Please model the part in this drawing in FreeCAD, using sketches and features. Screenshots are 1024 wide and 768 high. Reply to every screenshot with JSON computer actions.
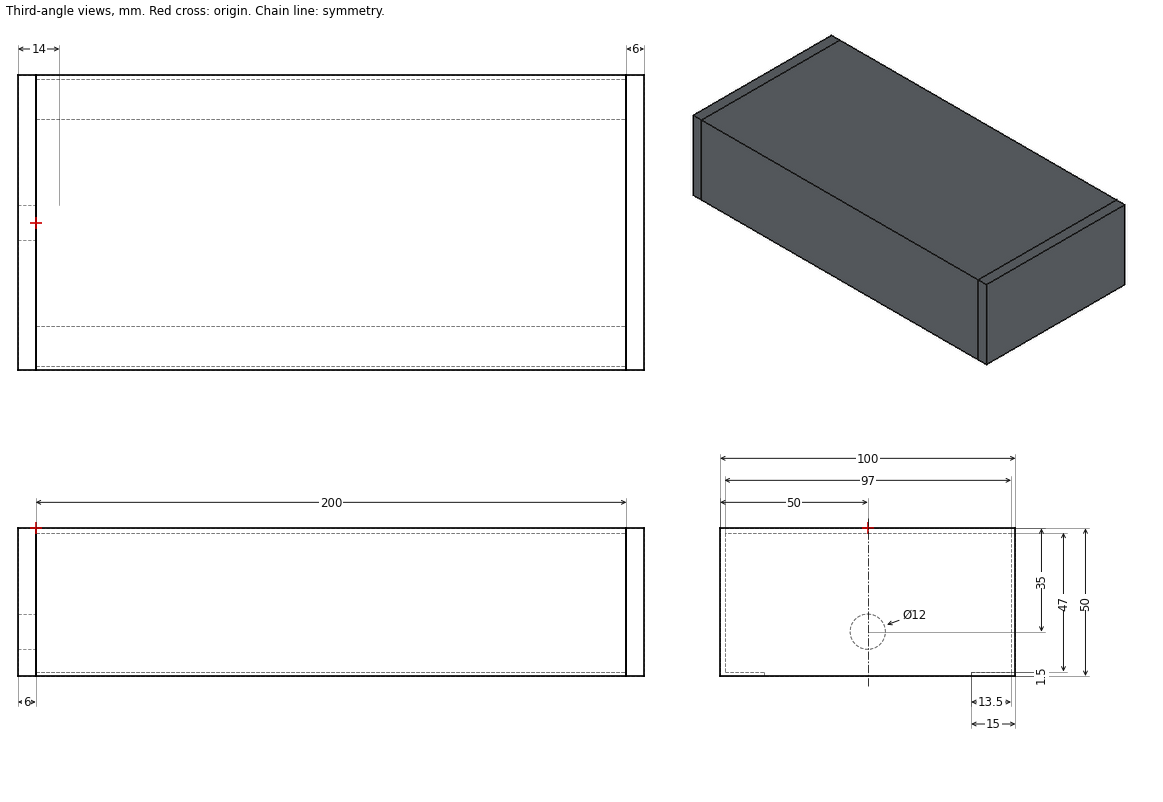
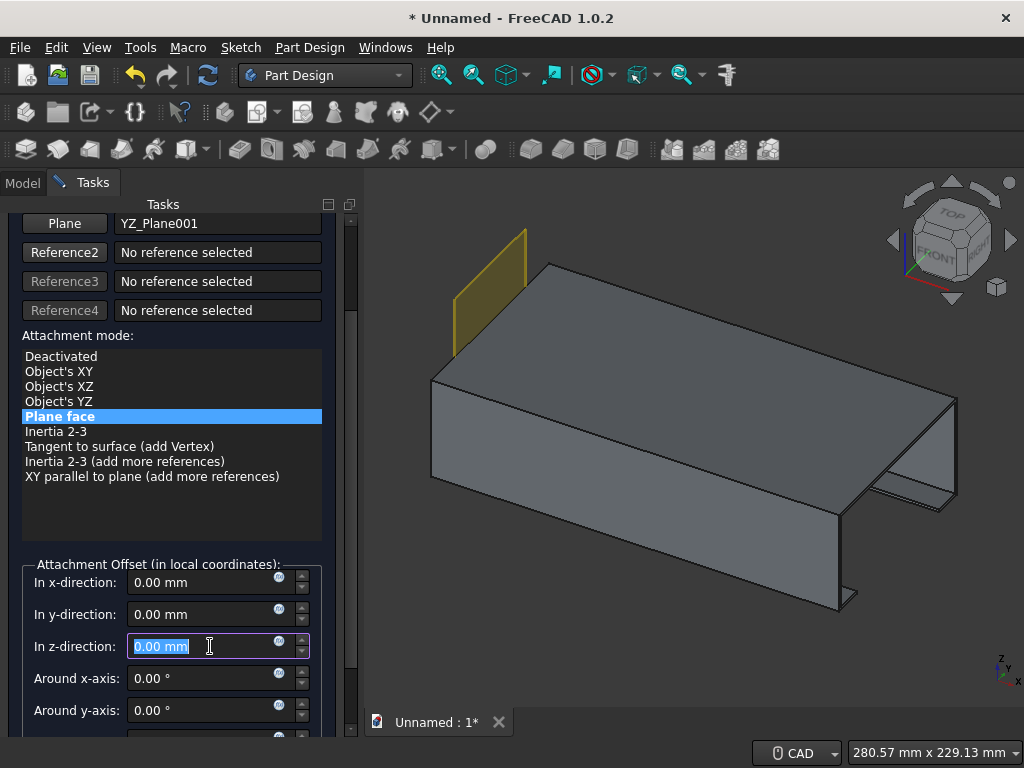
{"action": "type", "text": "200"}
{"action": "key", "text": "Tab"}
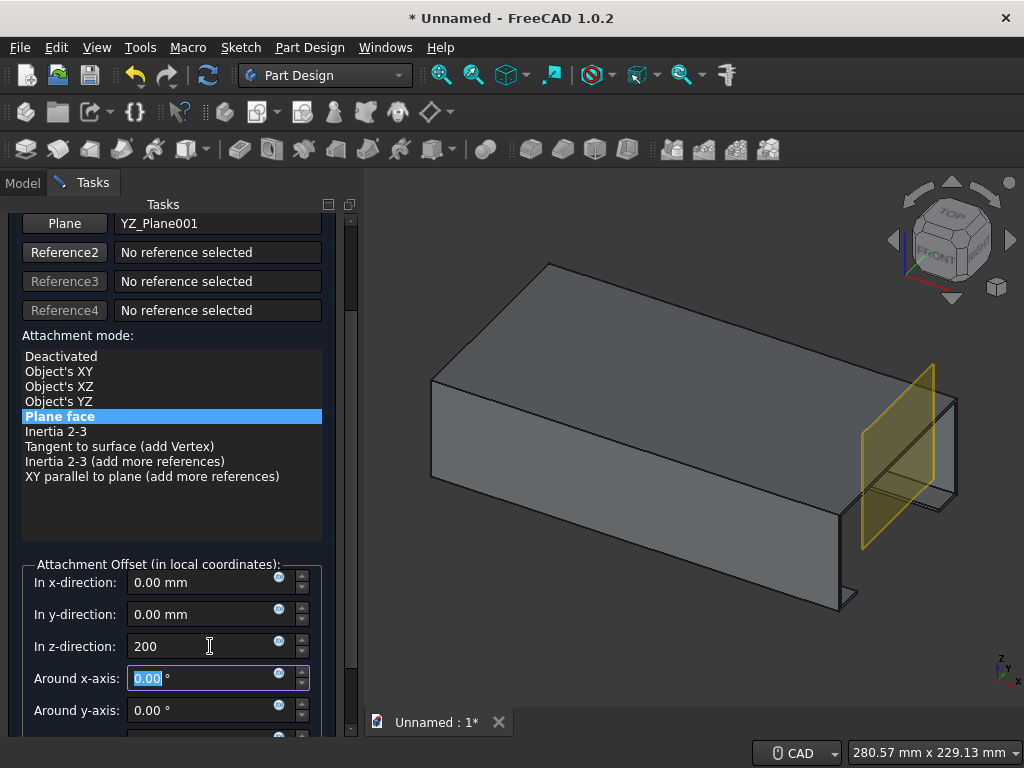
{"action": "scroll", "coordinate": [351, 475], "scroll_direction": "up", "scroll_amount": 3}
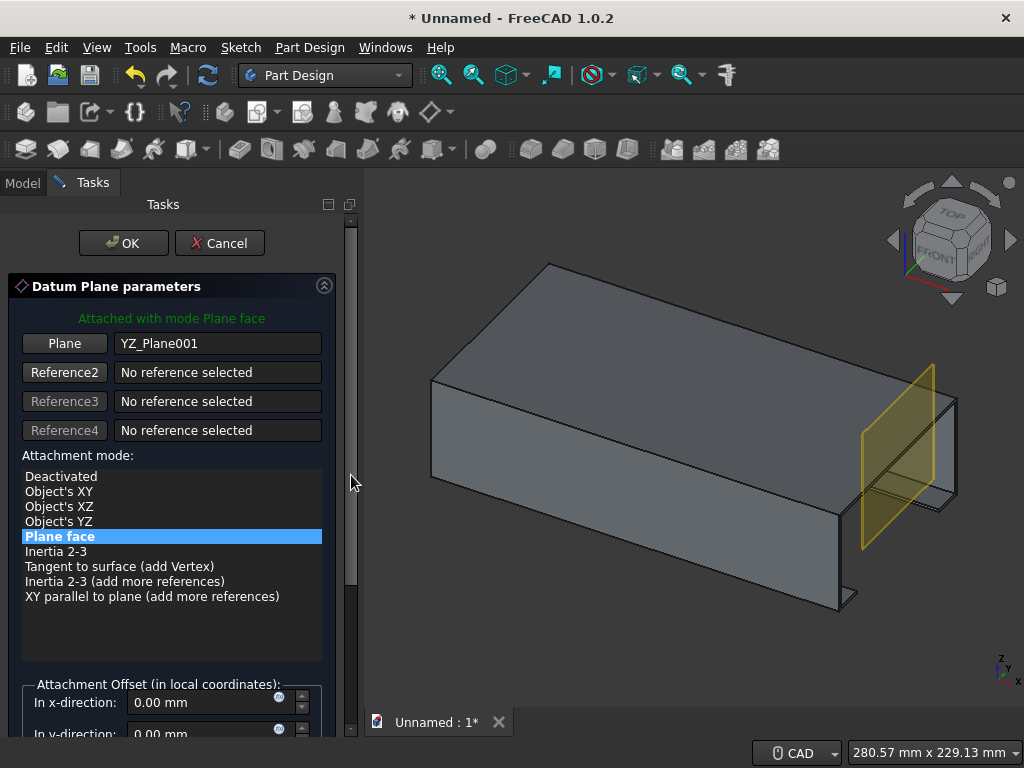
{"action": "left_click", "coordinate": [124, 243]}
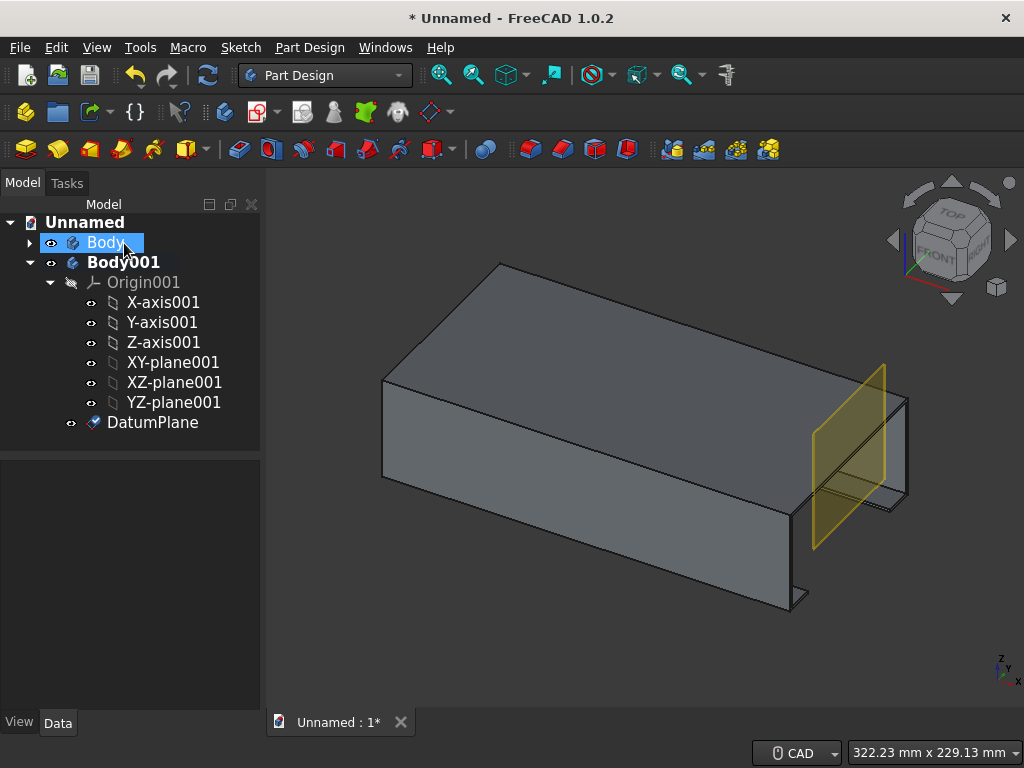
{"action": "left_click", "coordinate": [116, 423]}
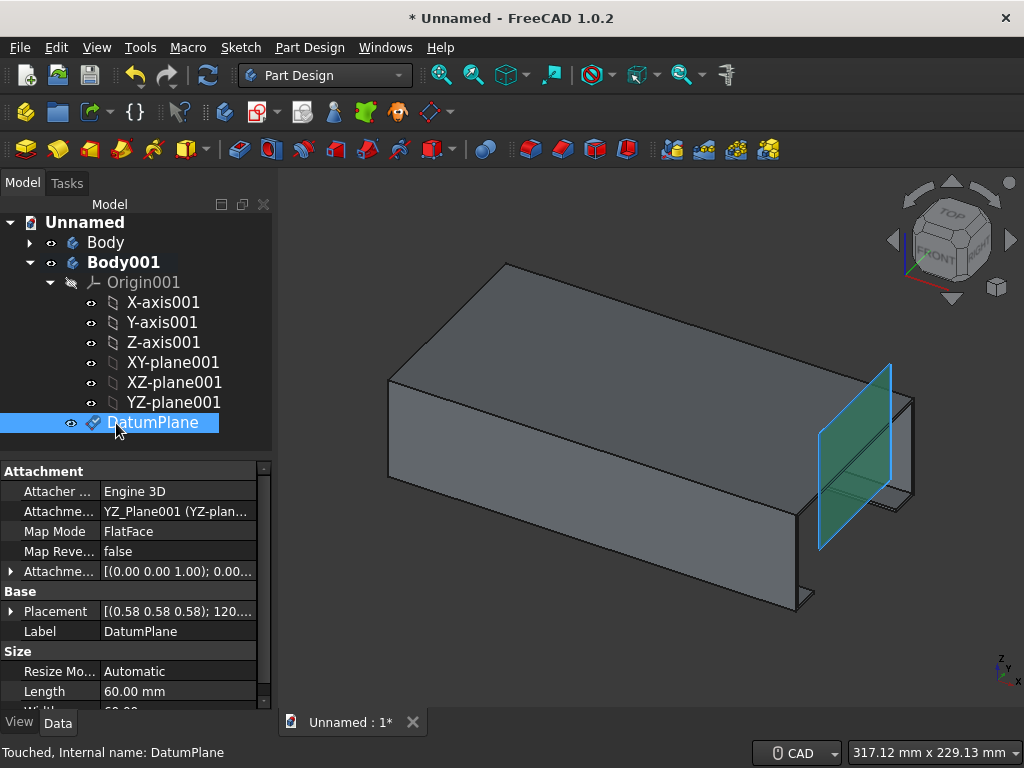
{"action": "left_click", "coordinate": [258, 112]}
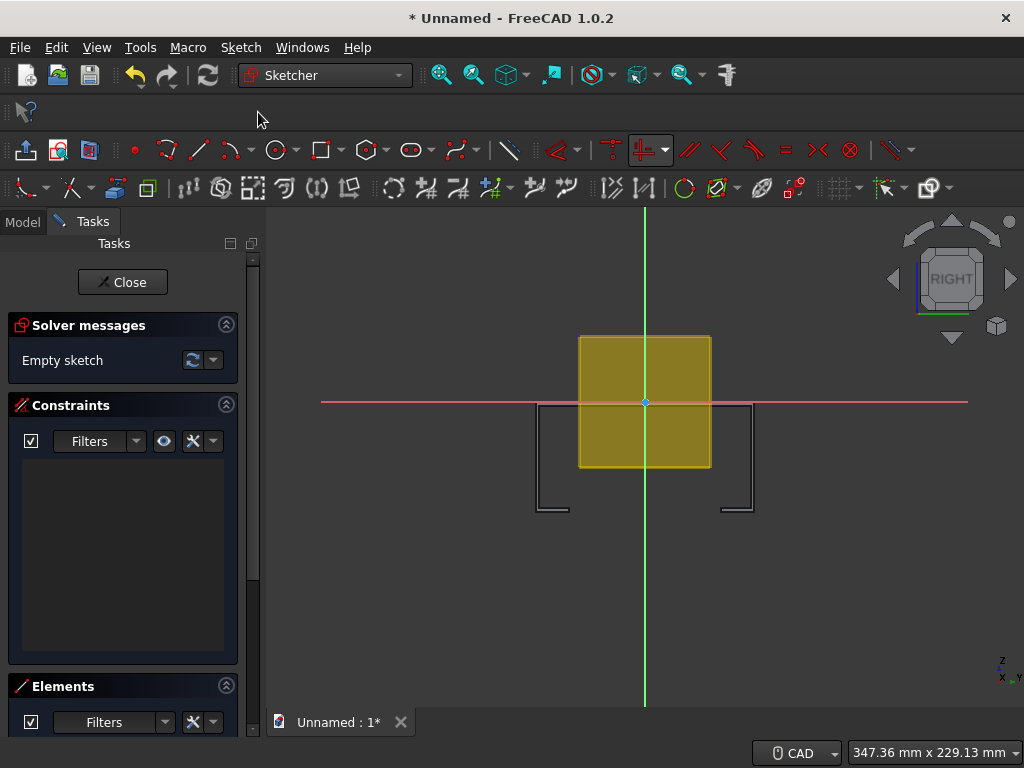
{"action": "scroll", "coordinate": [728, 457], "scroll_direction": "up", "scroll_amount": 3}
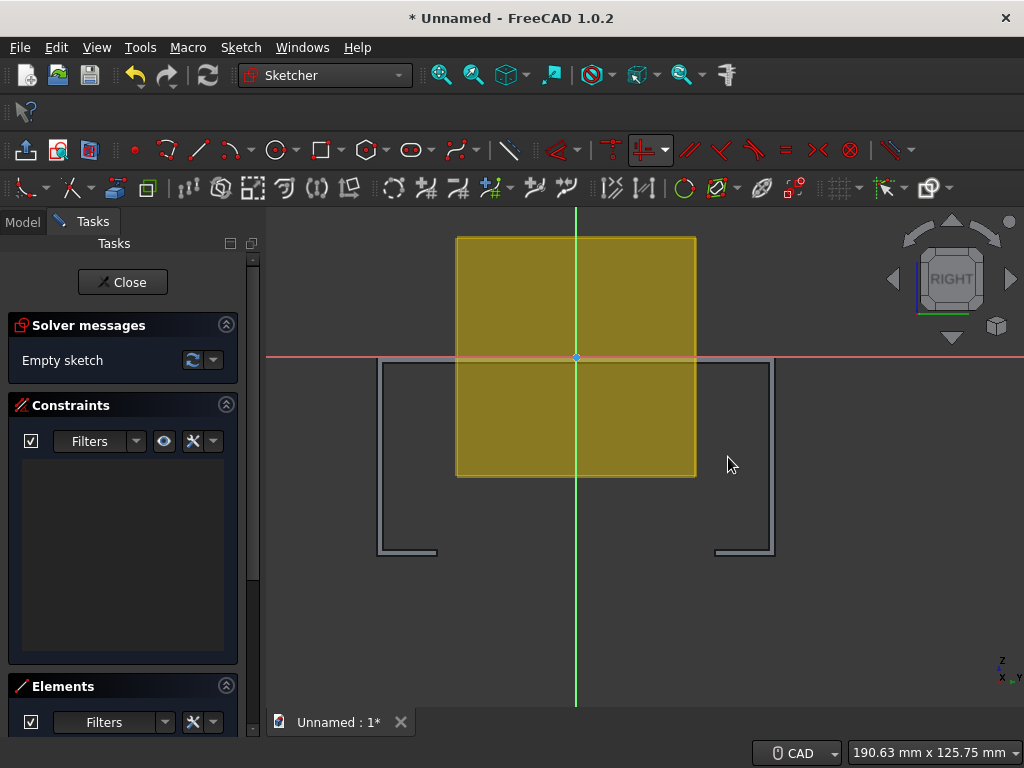
{"action": "left_click", "coordinate": [322, 150]}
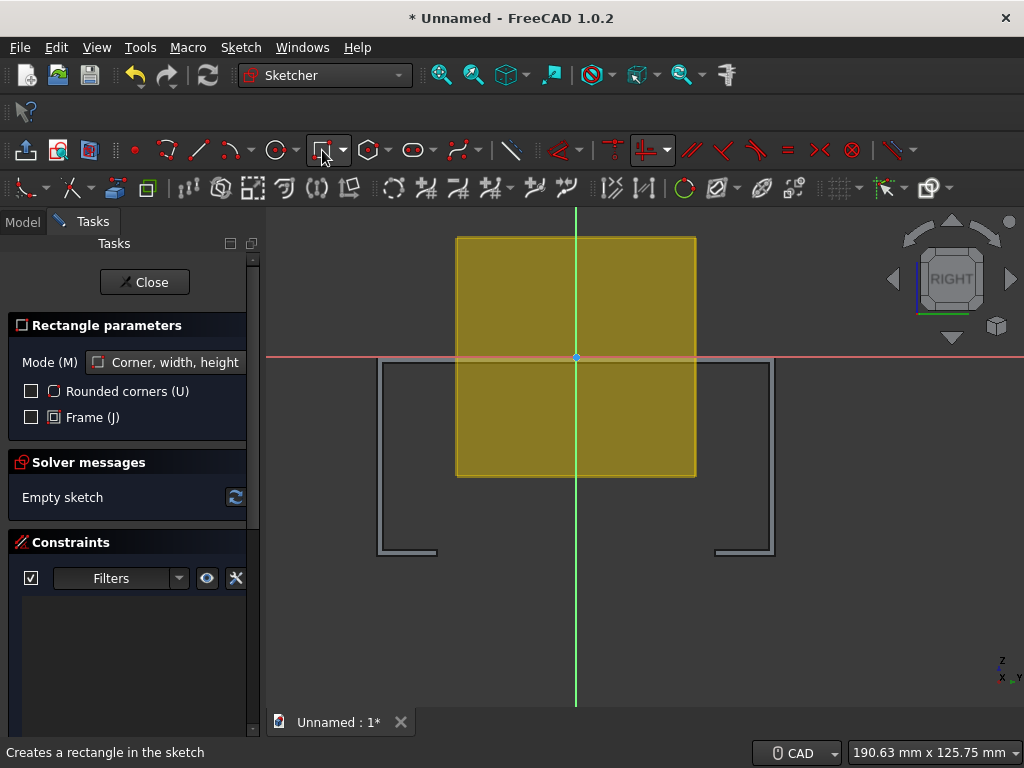
{"action": "left_click", "coordinate": [377, 357]}
{"action": "mouse_move", "coordinate": [775, 556]}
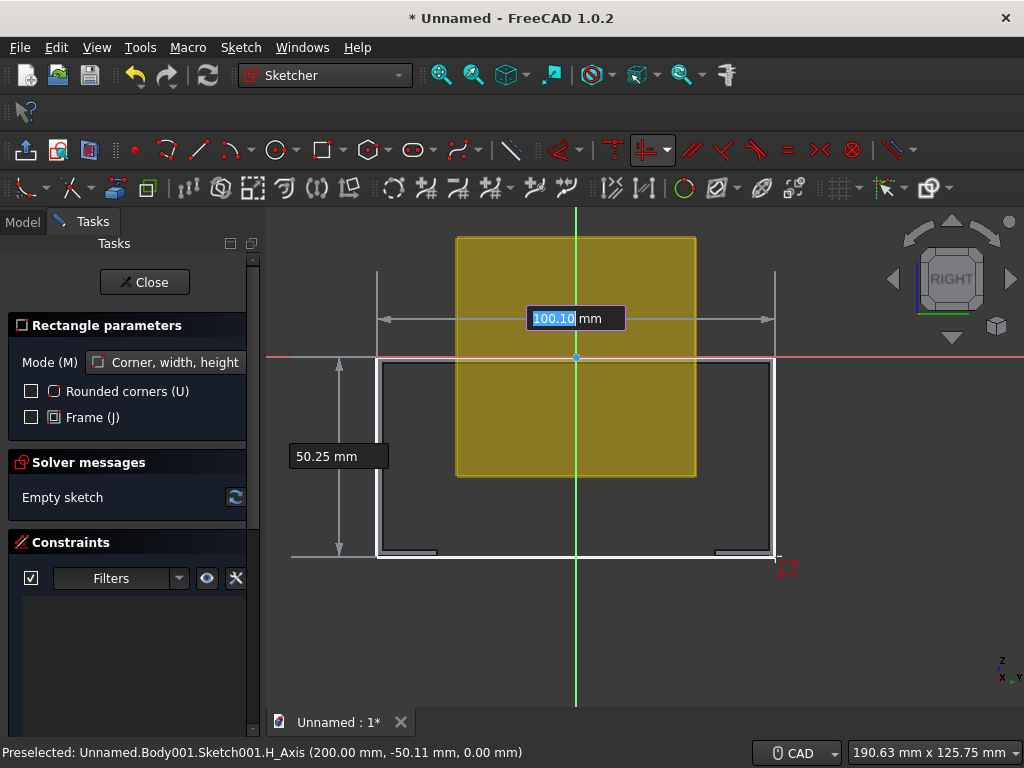
{"action": "type", "text": "100"}
{"action": "key", "text": "Tab"}
{"action": "type", "text": "50"}
{"action": "key", "text": "Return"}
{"action": "key", "text": "Escape"}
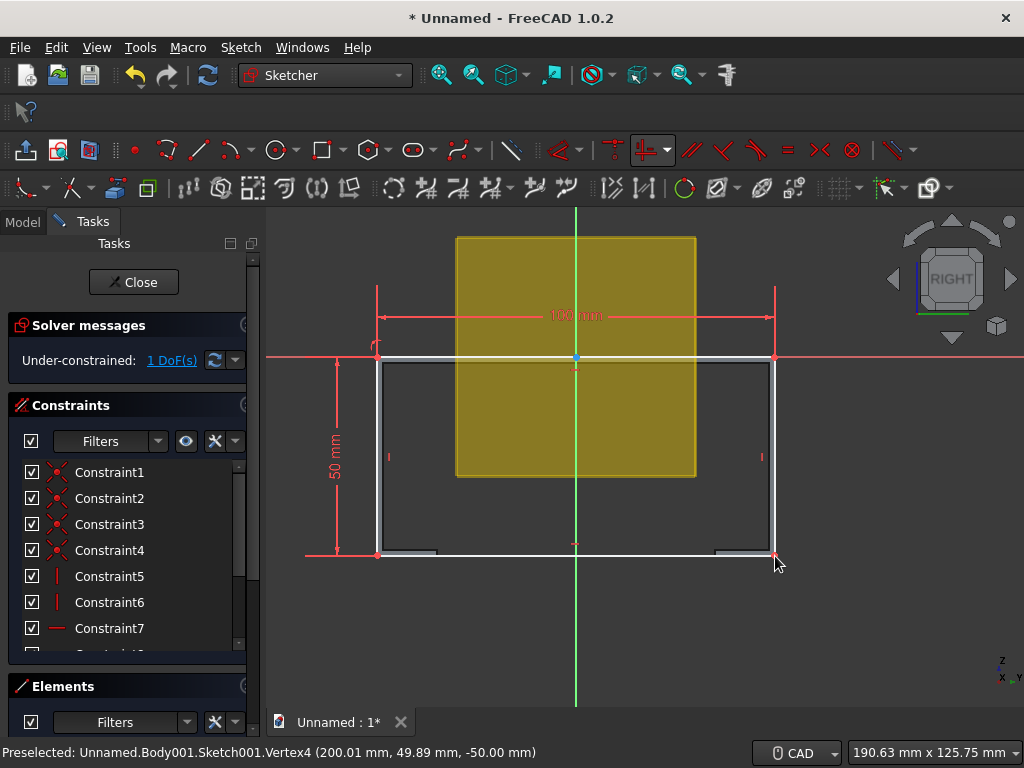
{"action": "left_click", "coordinate": [558, 150]}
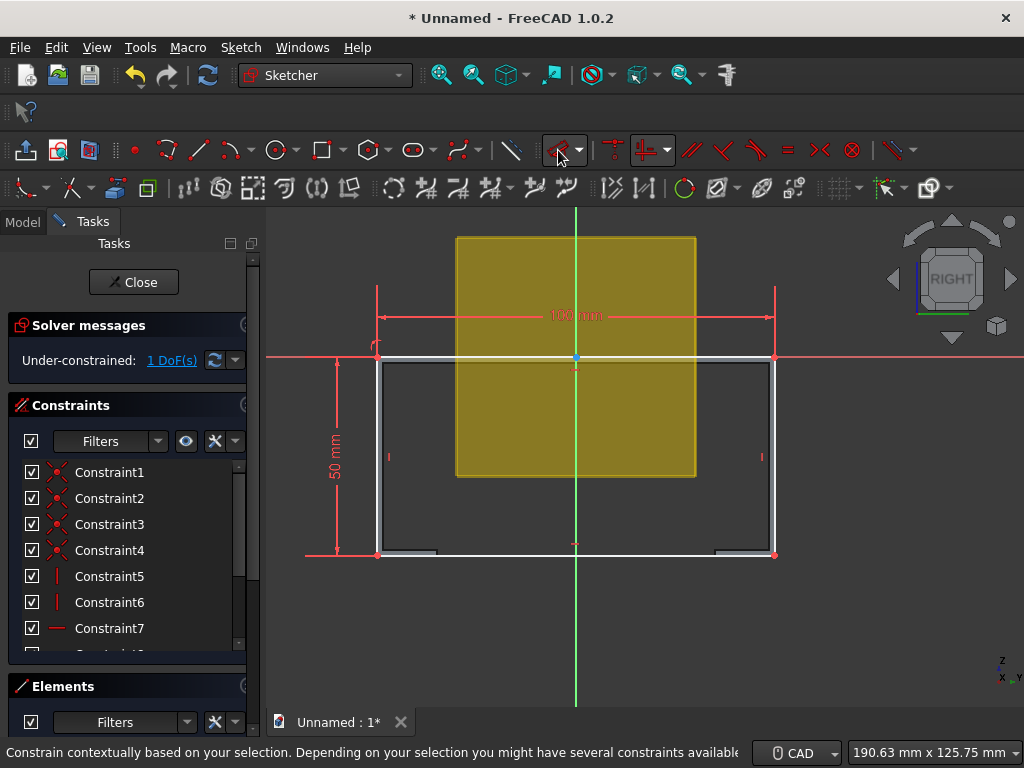
{"action": "left_click", "coordinate": [377, 357]}
{"action": "left_click", "coordinate": [477, 323]}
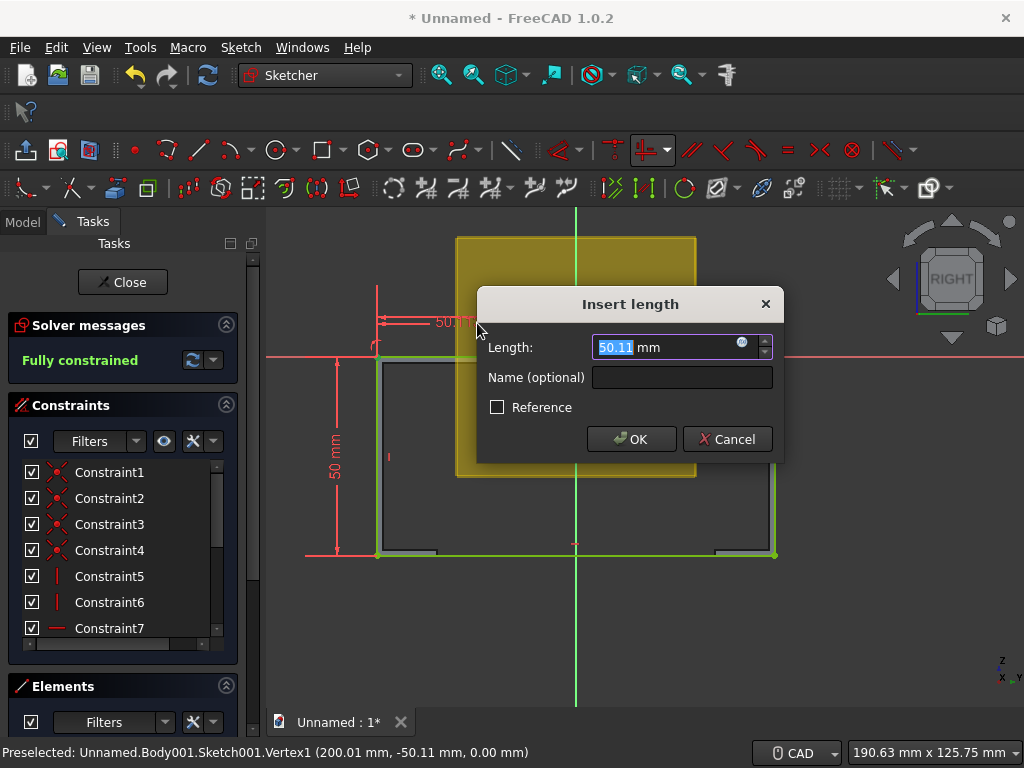
{"action": "type", "text": "50"}
{"action": "key", "text": "Return"}
{"action": "key", "text": "Escape"}